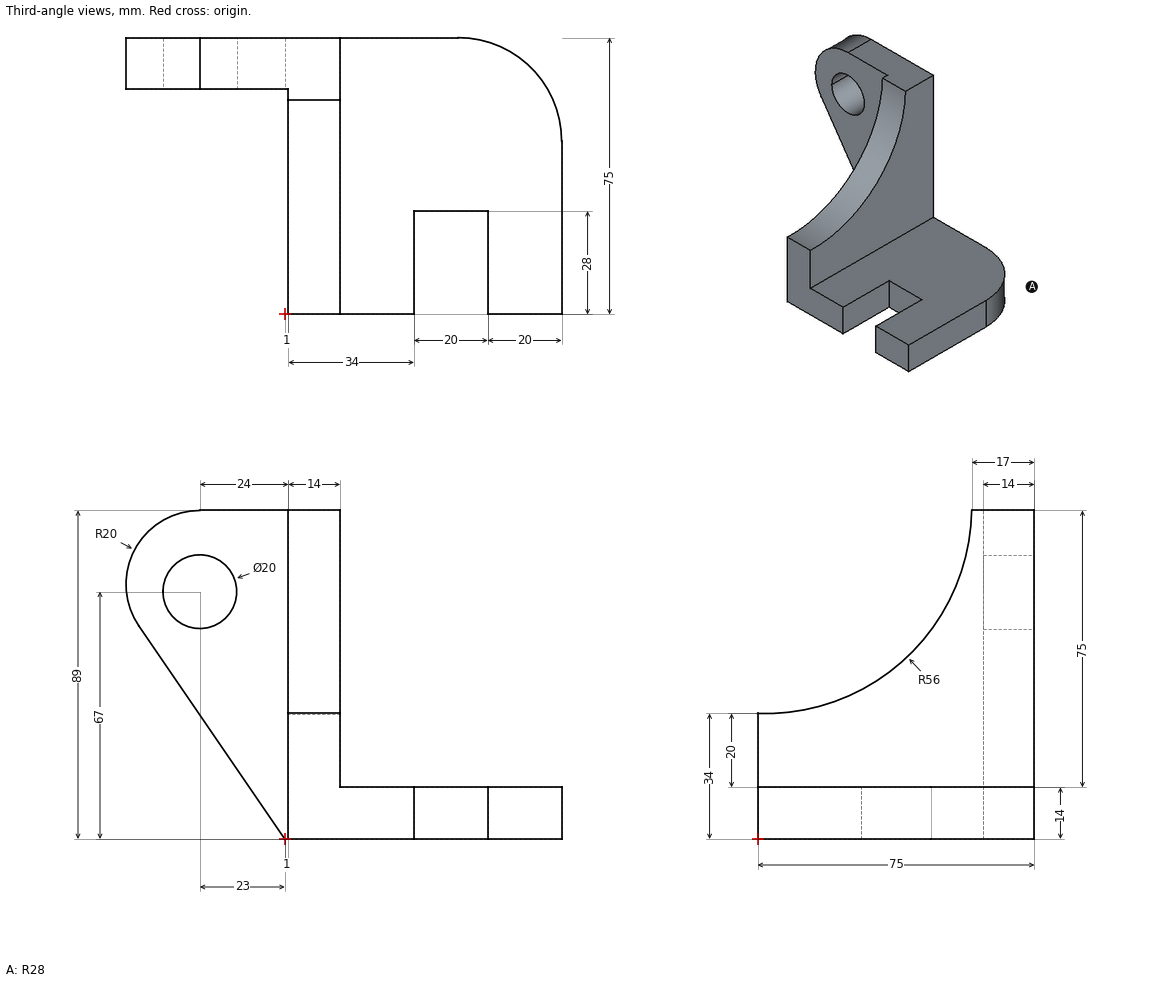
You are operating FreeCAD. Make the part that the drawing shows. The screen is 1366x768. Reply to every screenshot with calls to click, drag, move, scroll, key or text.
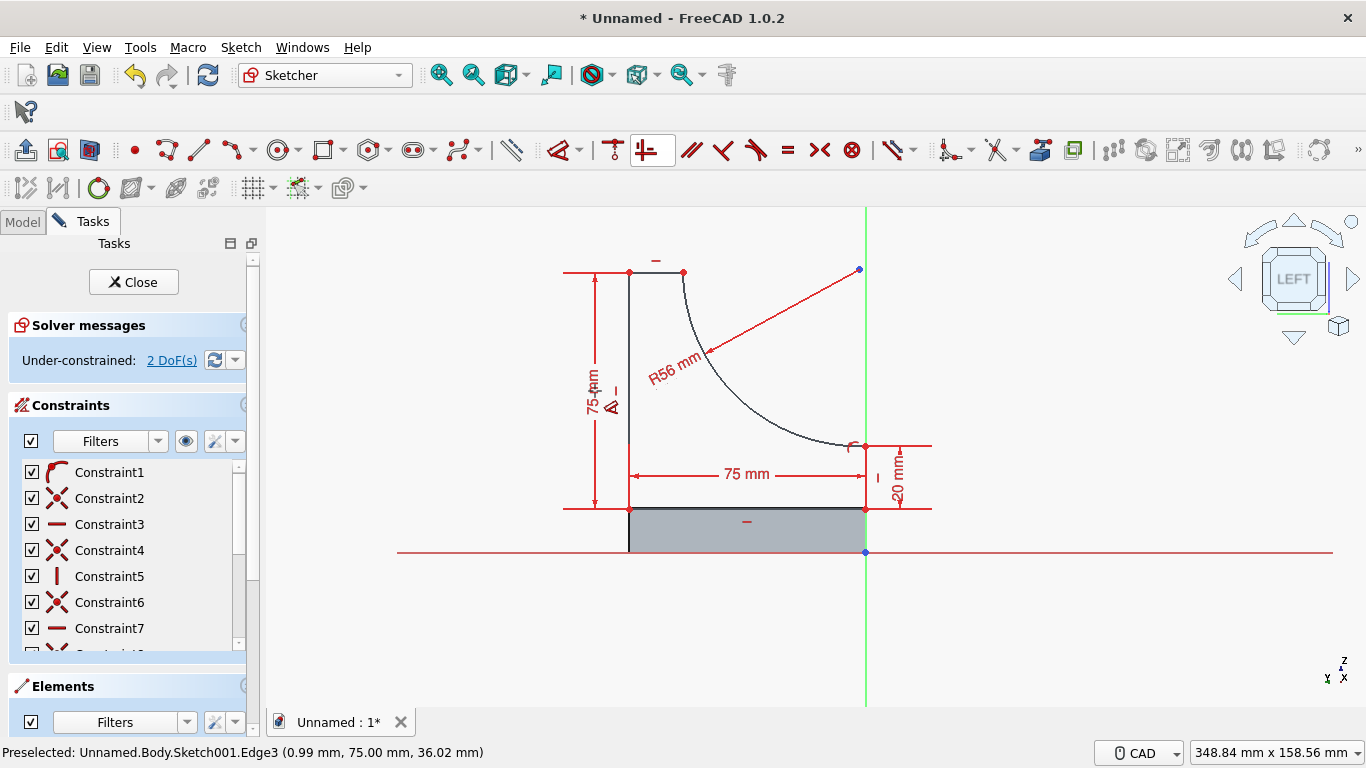
click(645, 273)
click(656, 239)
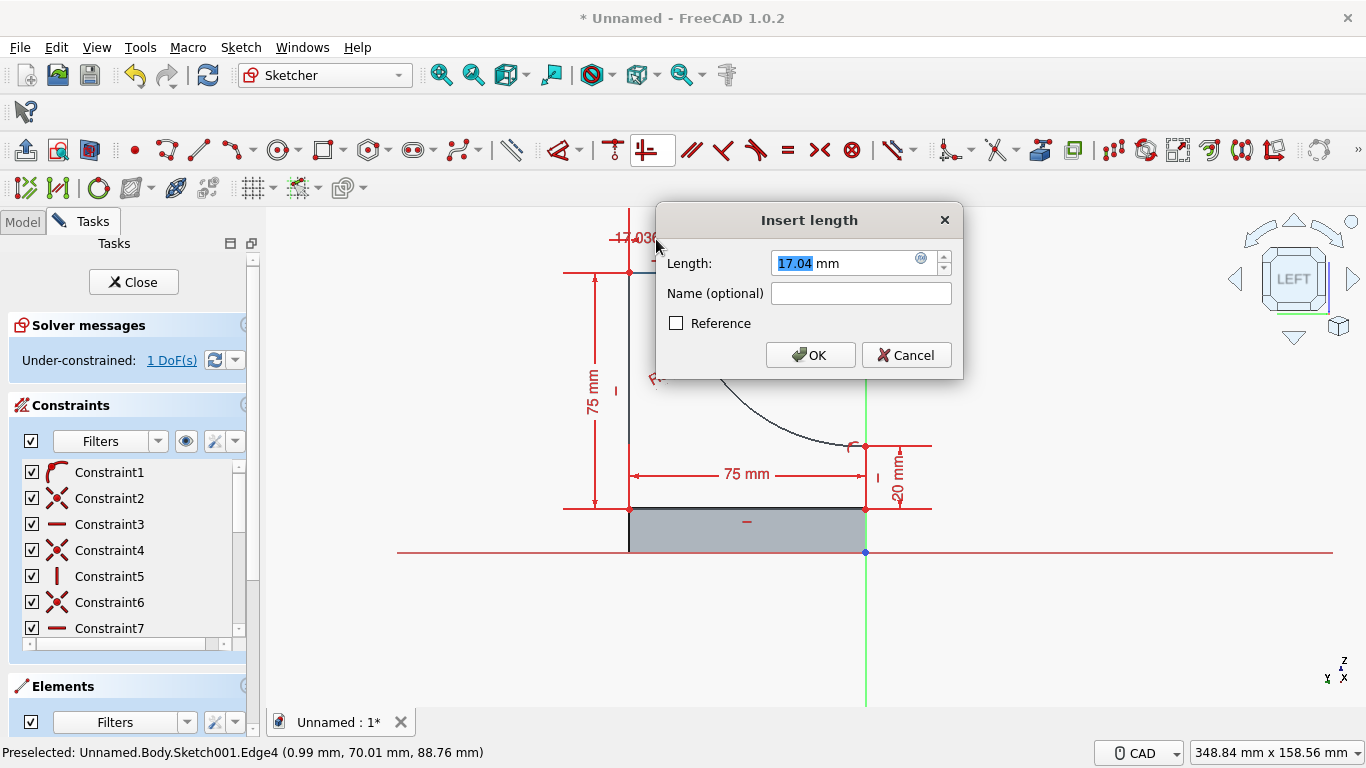
text(17)
key(Return)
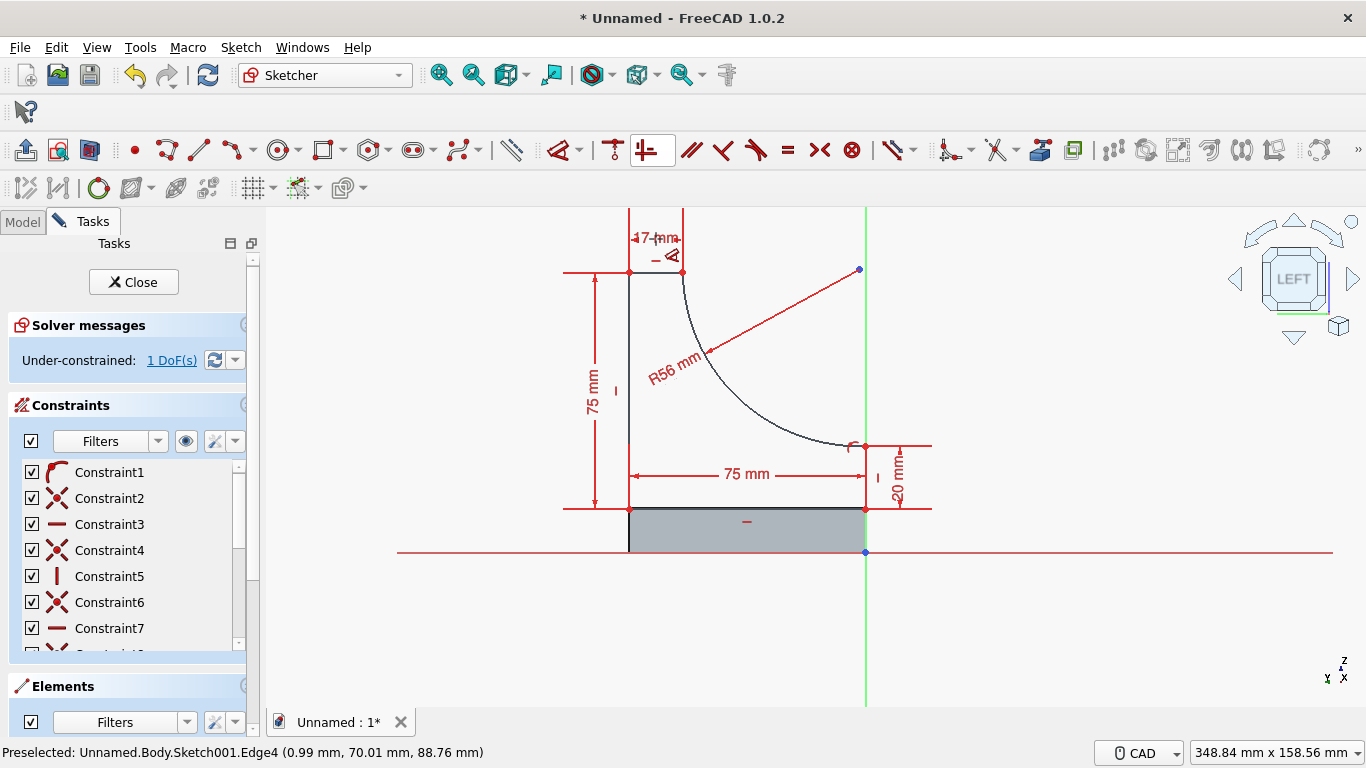
click(866, 446)
click(900, 499)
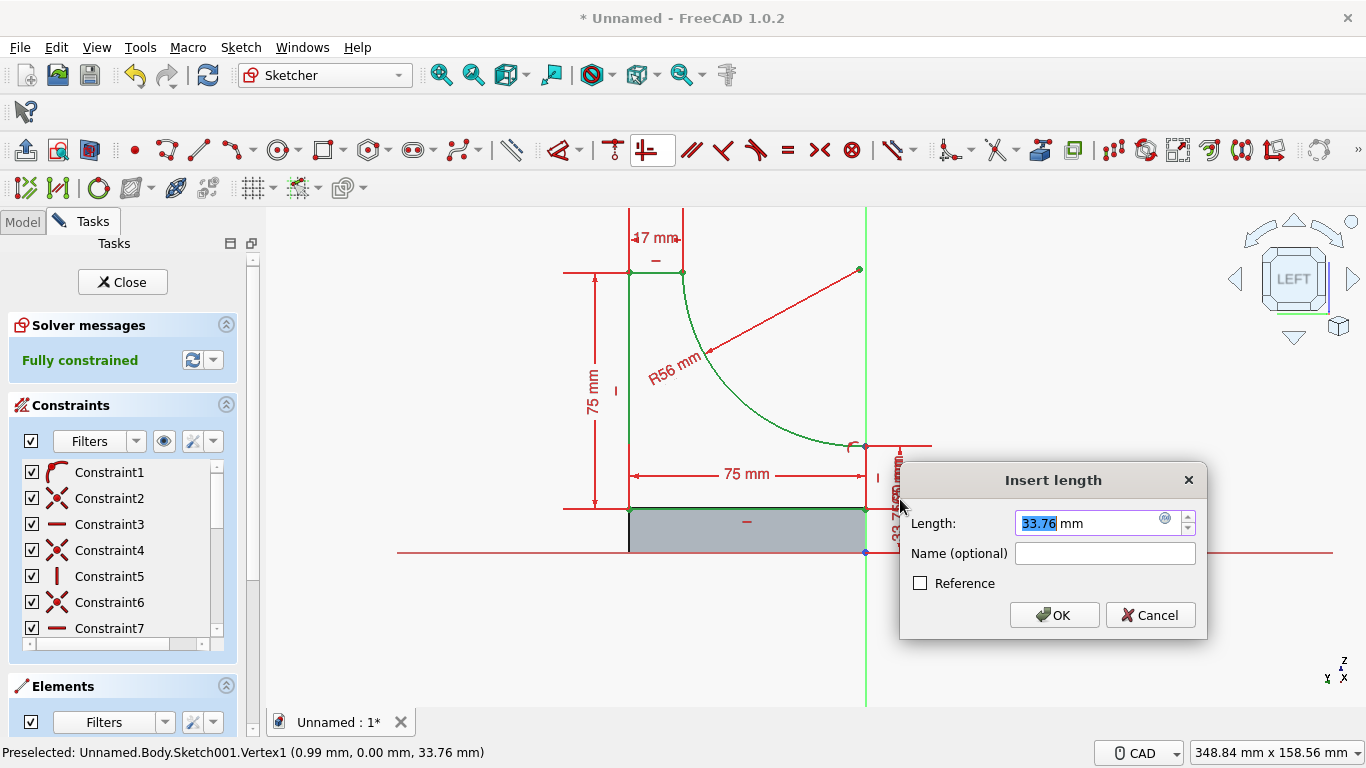
text(34)
key(Return)
key(Escape)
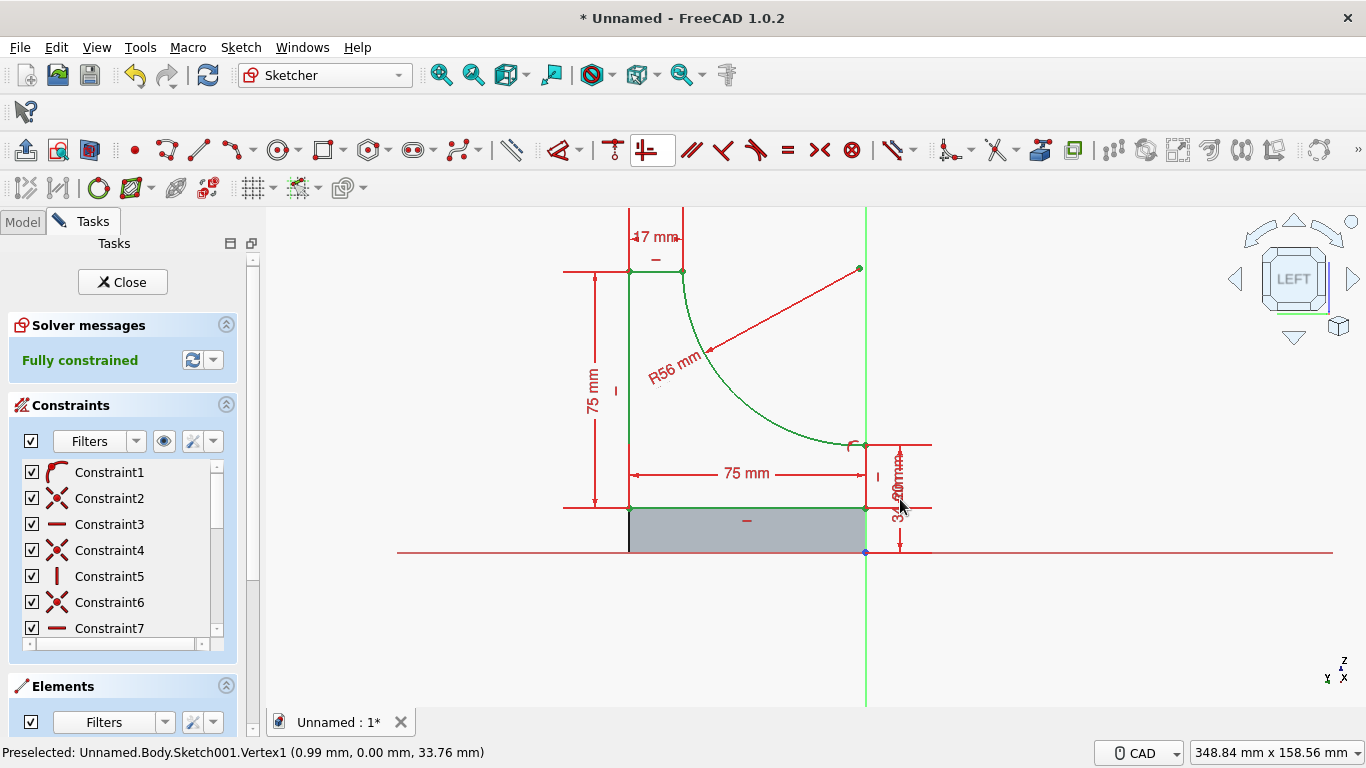
click(123, 282)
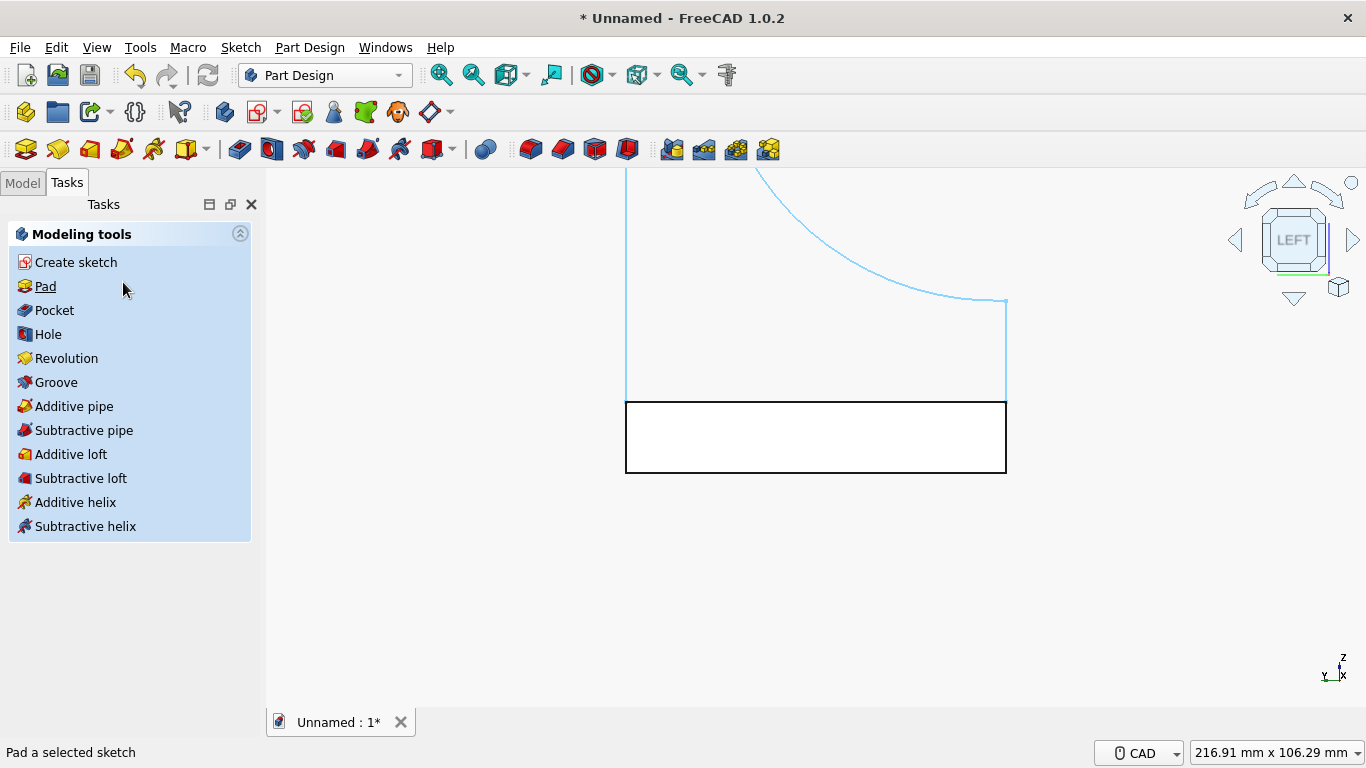
click(26, 150)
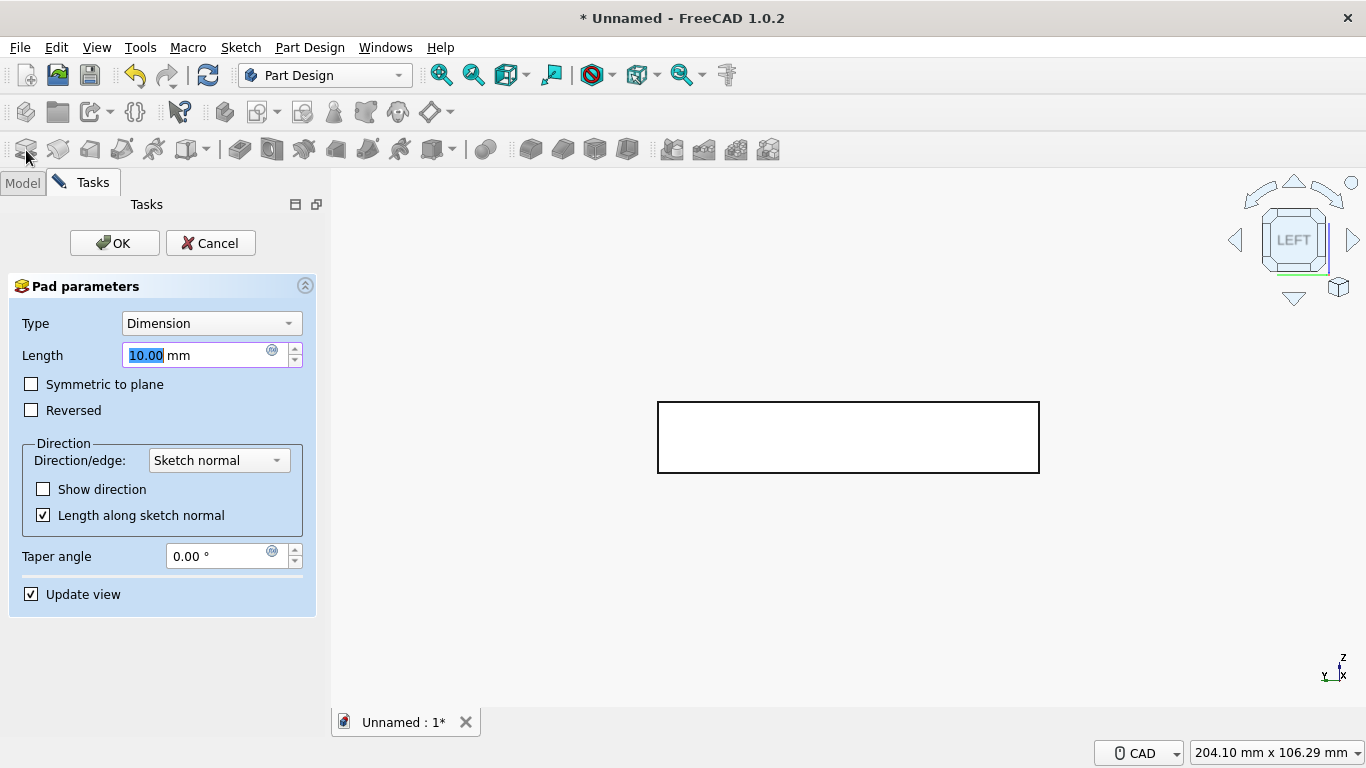
text(14)
key(Tab)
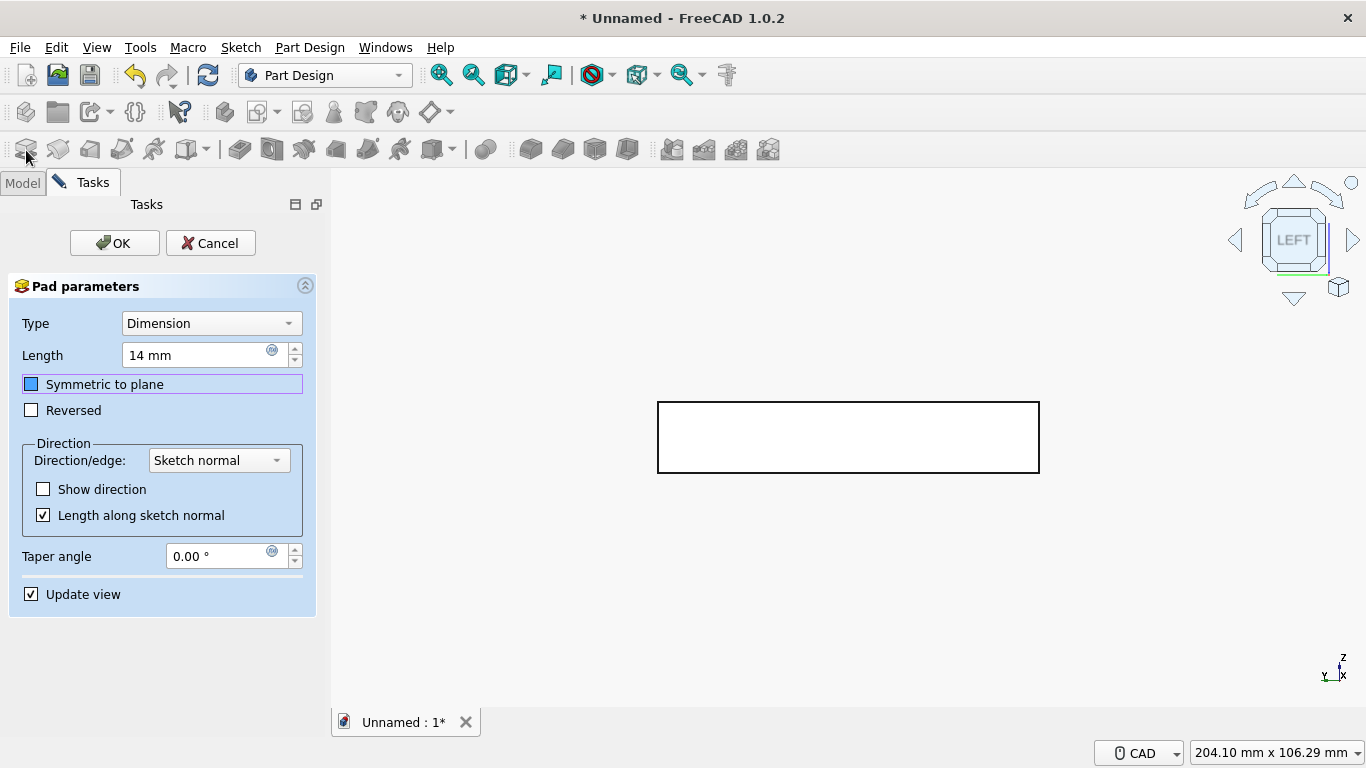
click(30, 410)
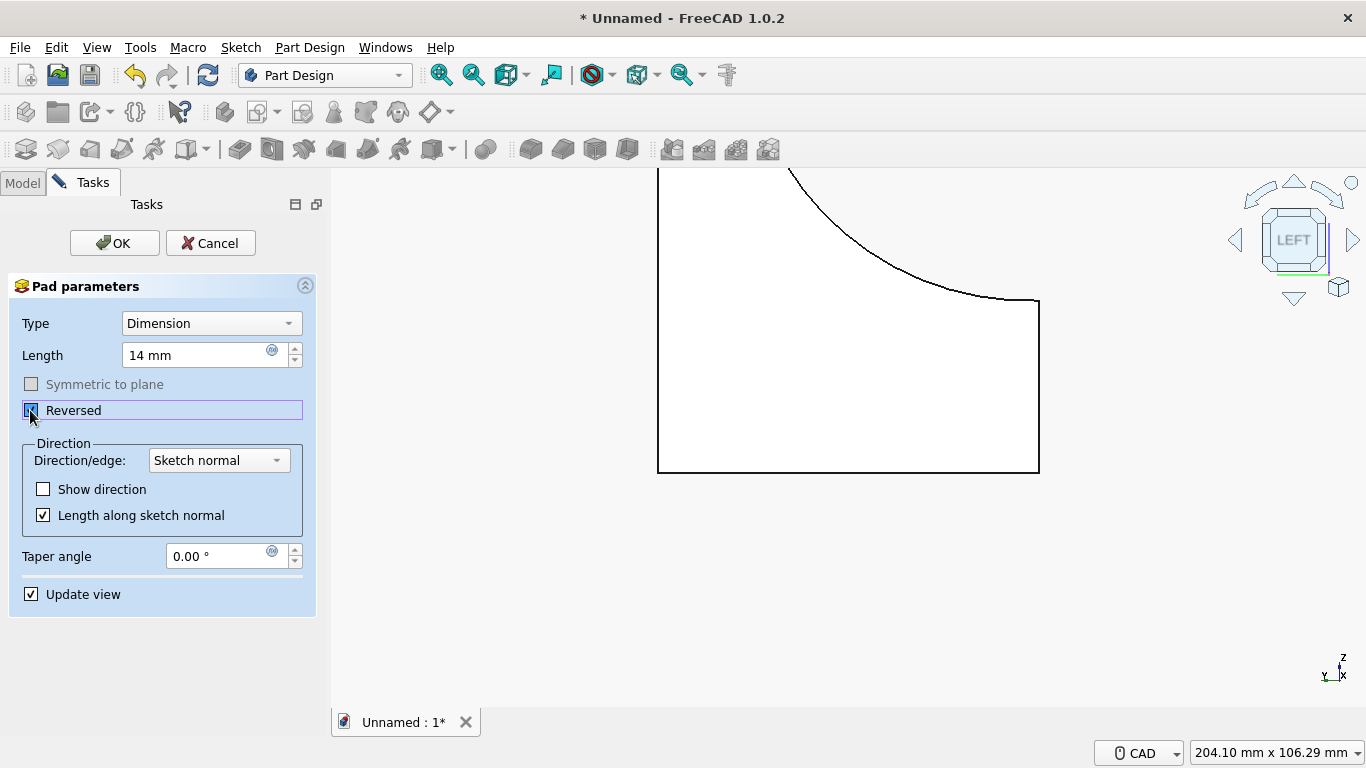
click(115, 243)